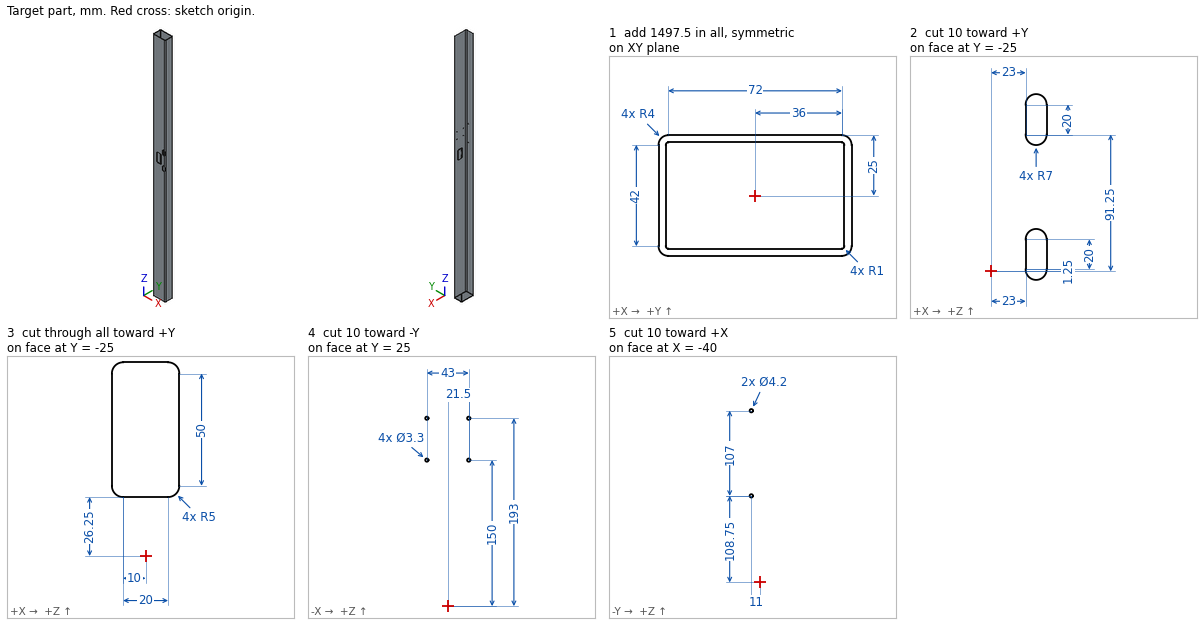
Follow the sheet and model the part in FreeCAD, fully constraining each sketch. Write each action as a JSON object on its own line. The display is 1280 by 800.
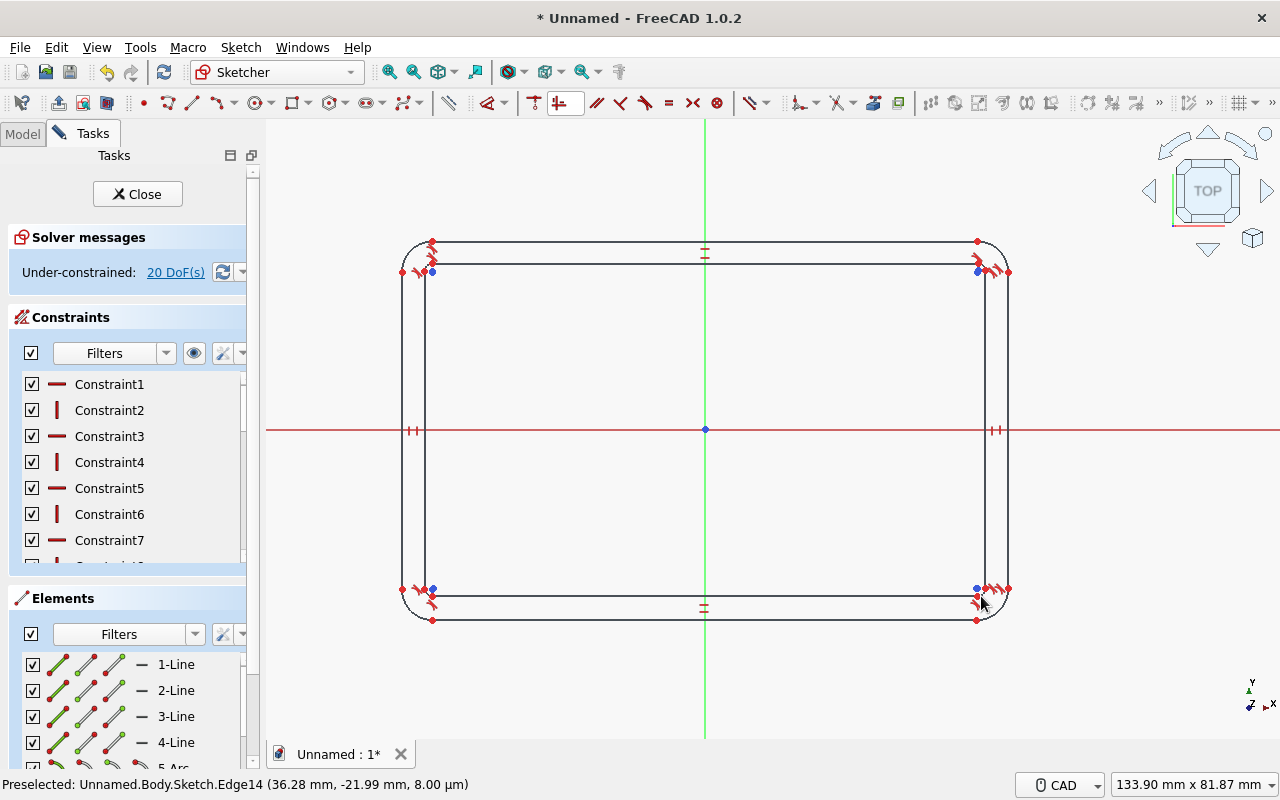
{"action": "left_click", "coordinate": [814, 596]}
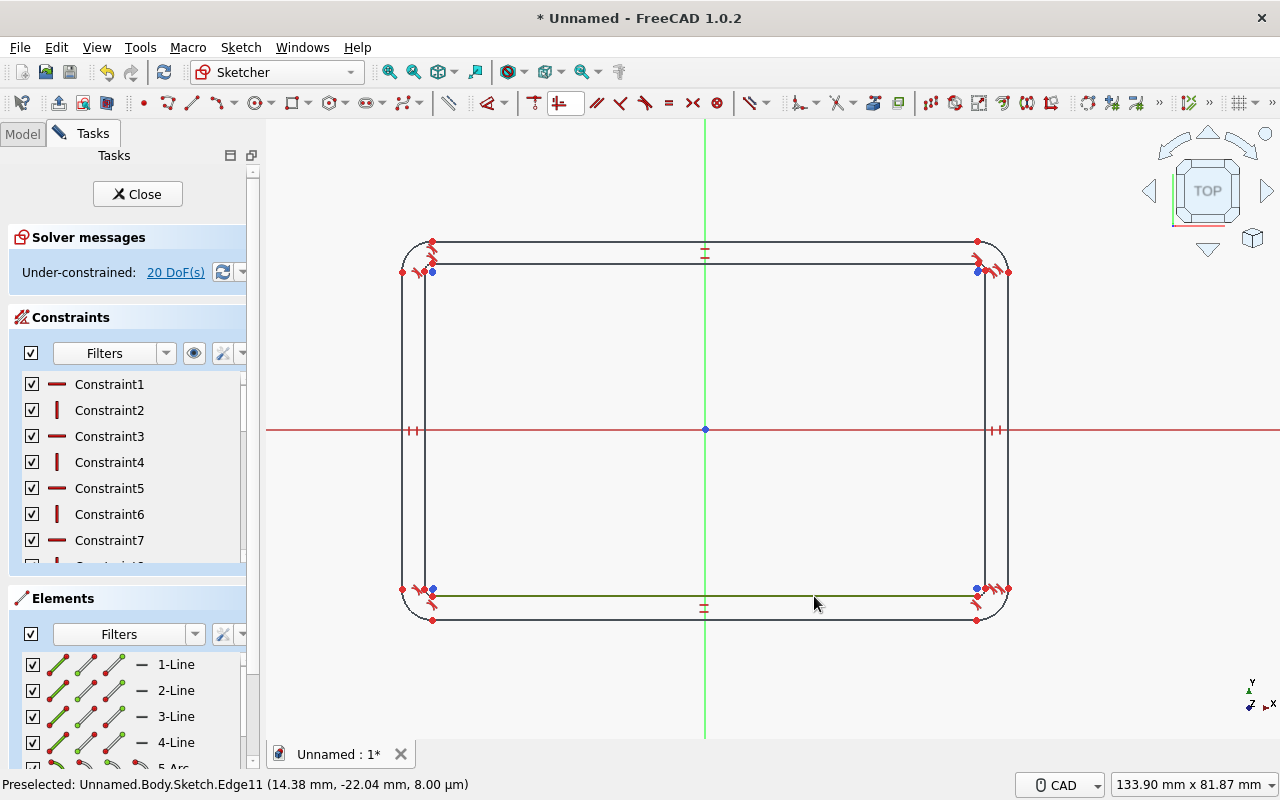
{"action": "scroll", "coordinate": [983, 594], "scroll_direction": "up", "scroll_amount": 5}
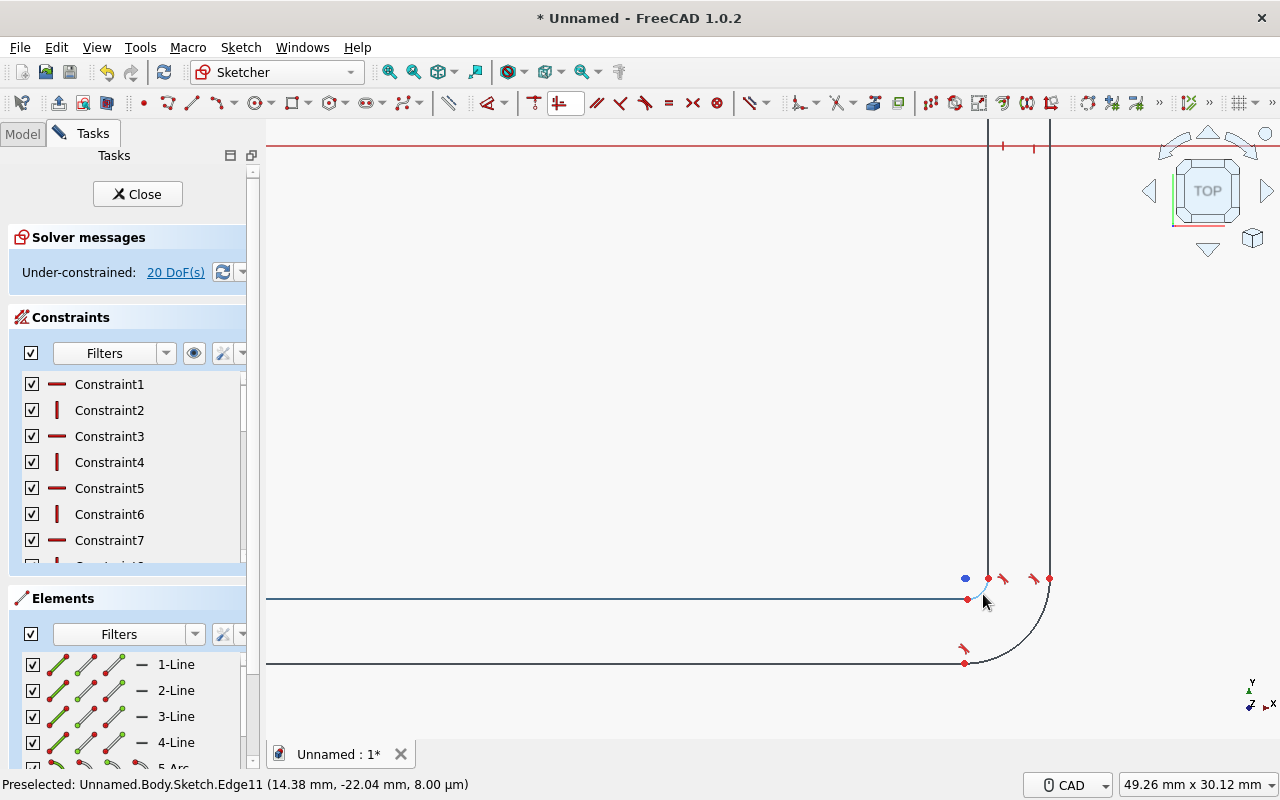
{"action": "left_click", "coordinate": [982, 593]}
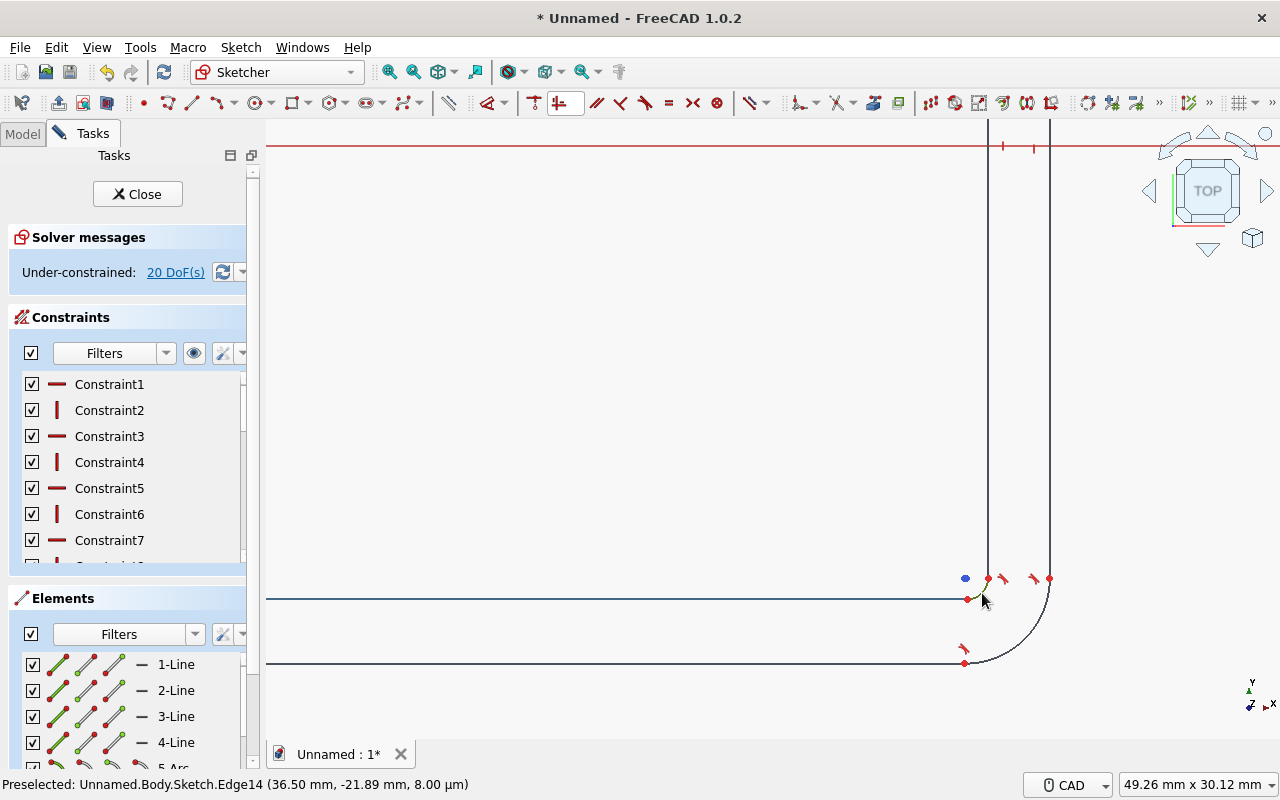
{"action": "key", "text": "t"}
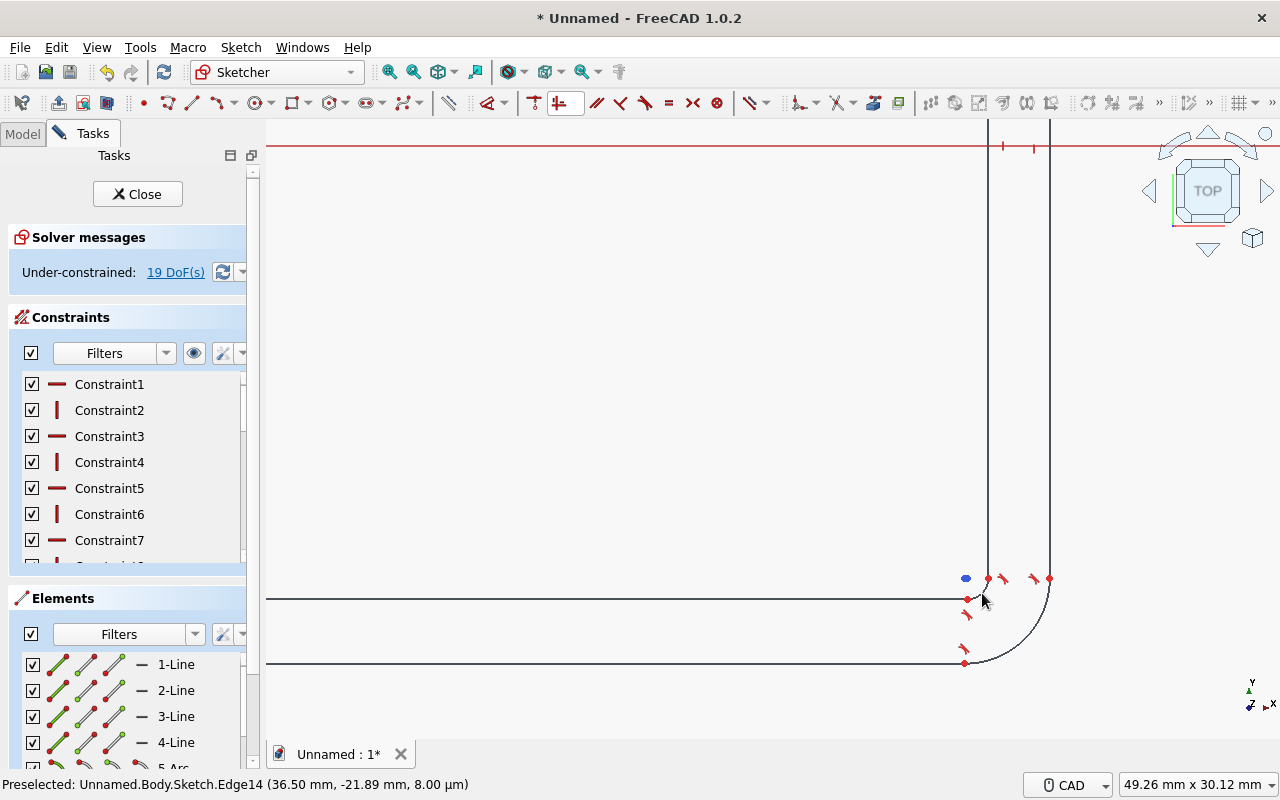
{"action": "left_click", "coordinate": [522, 599]}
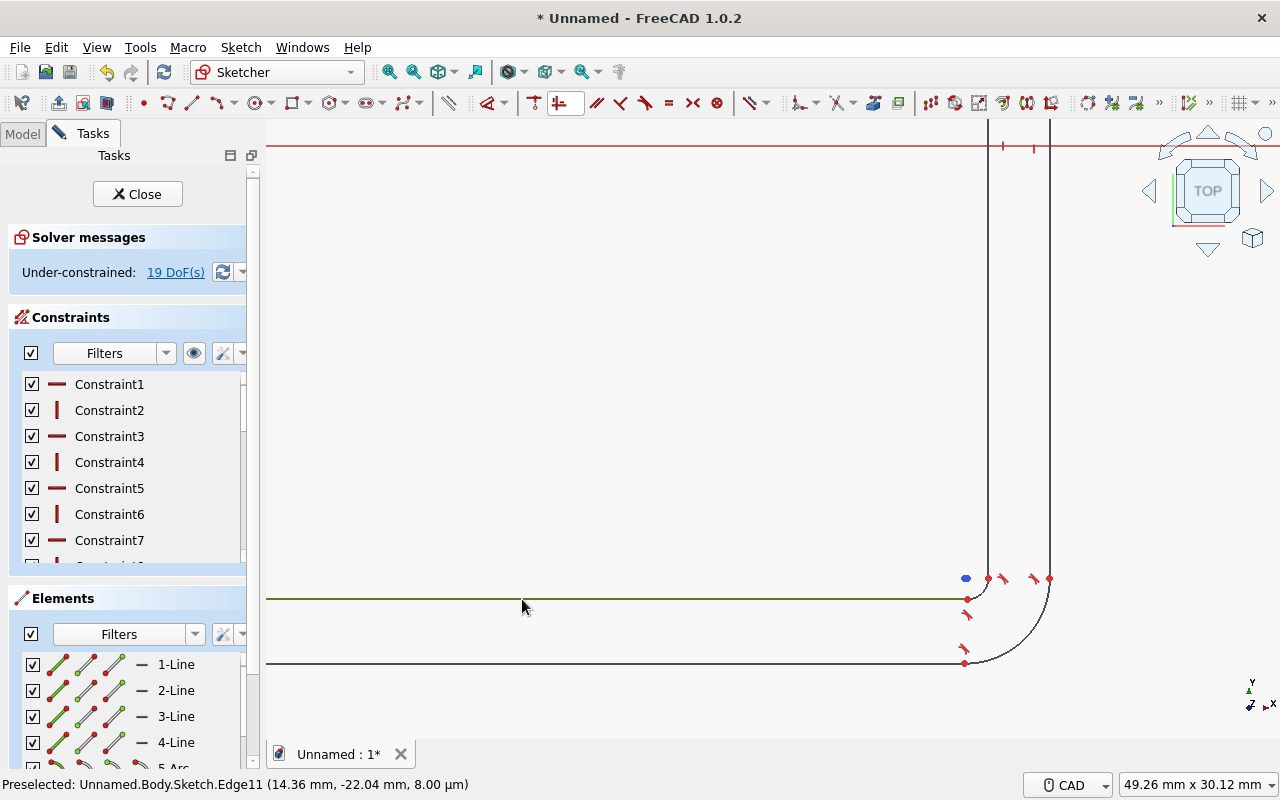
{"action": "scroll", "coordinate": [983, 594], "scroll_direction": "down", "scroll_amount": 5}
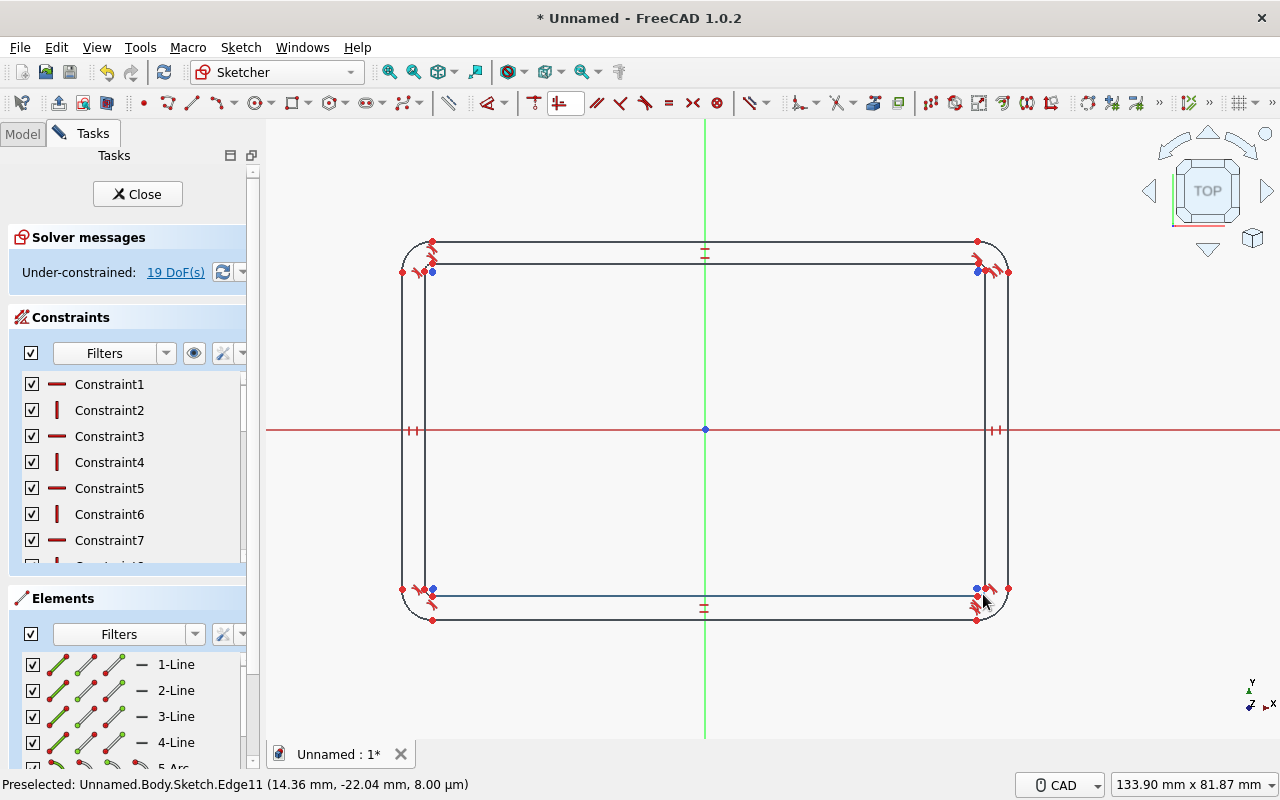
{"action": "scroll", "coordinate": [426, 592], "scroll_direction": "up", "scroll_amount": 8}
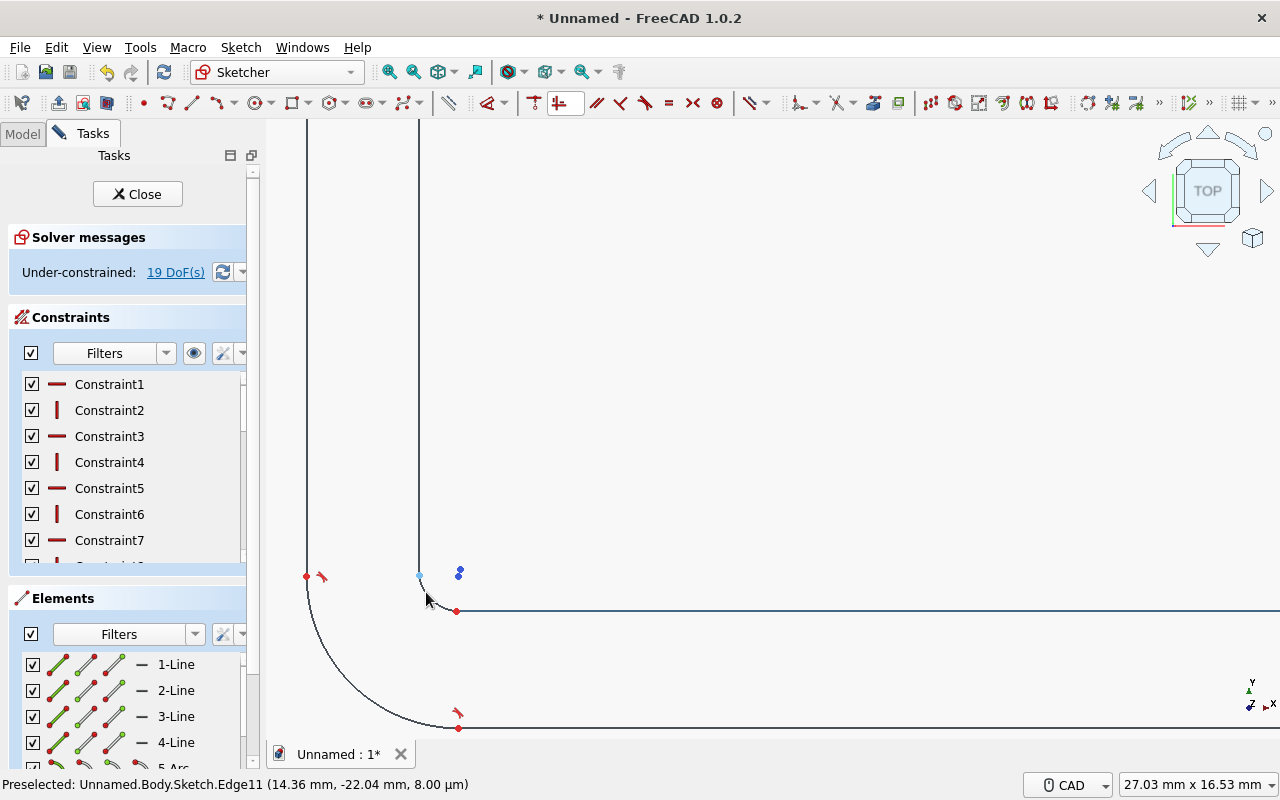
{"action": "left_click", "coordinate": [425, 591]}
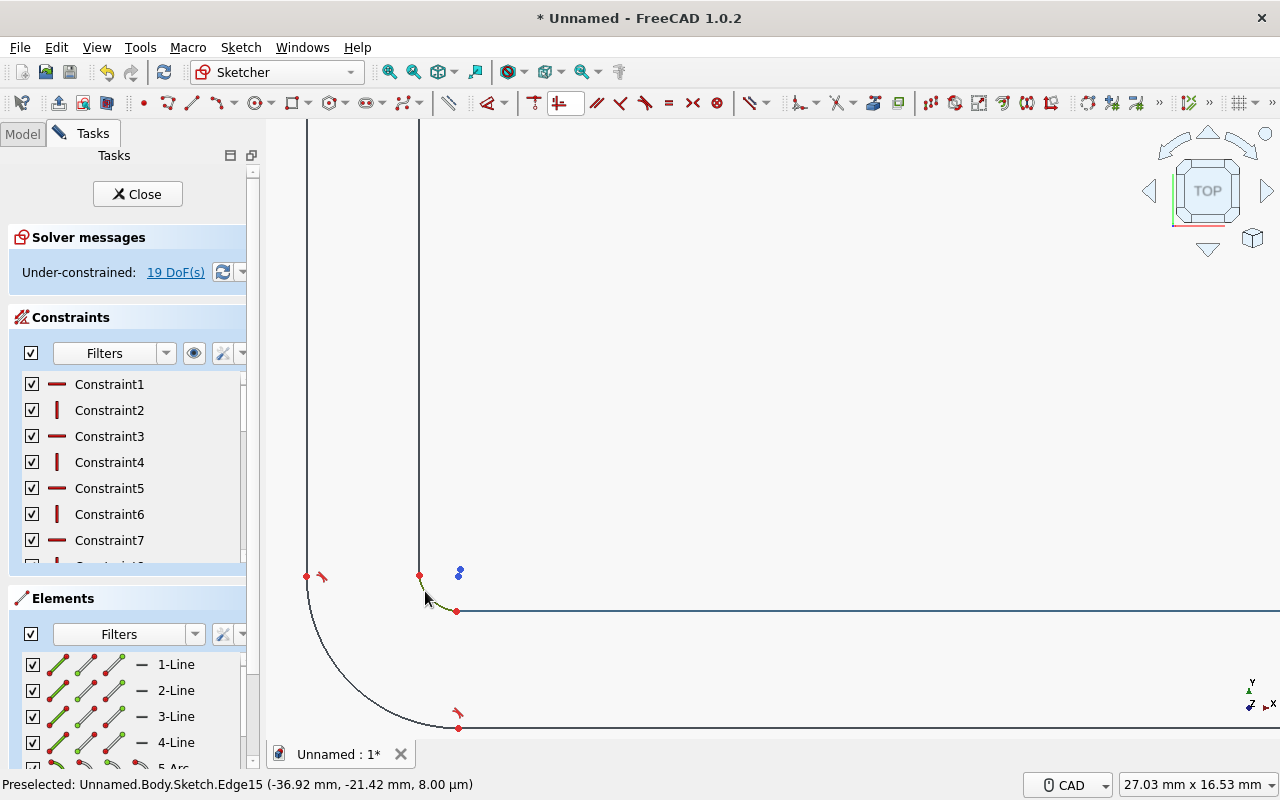
{"action": "left_click", "coordinate": [646, 104]}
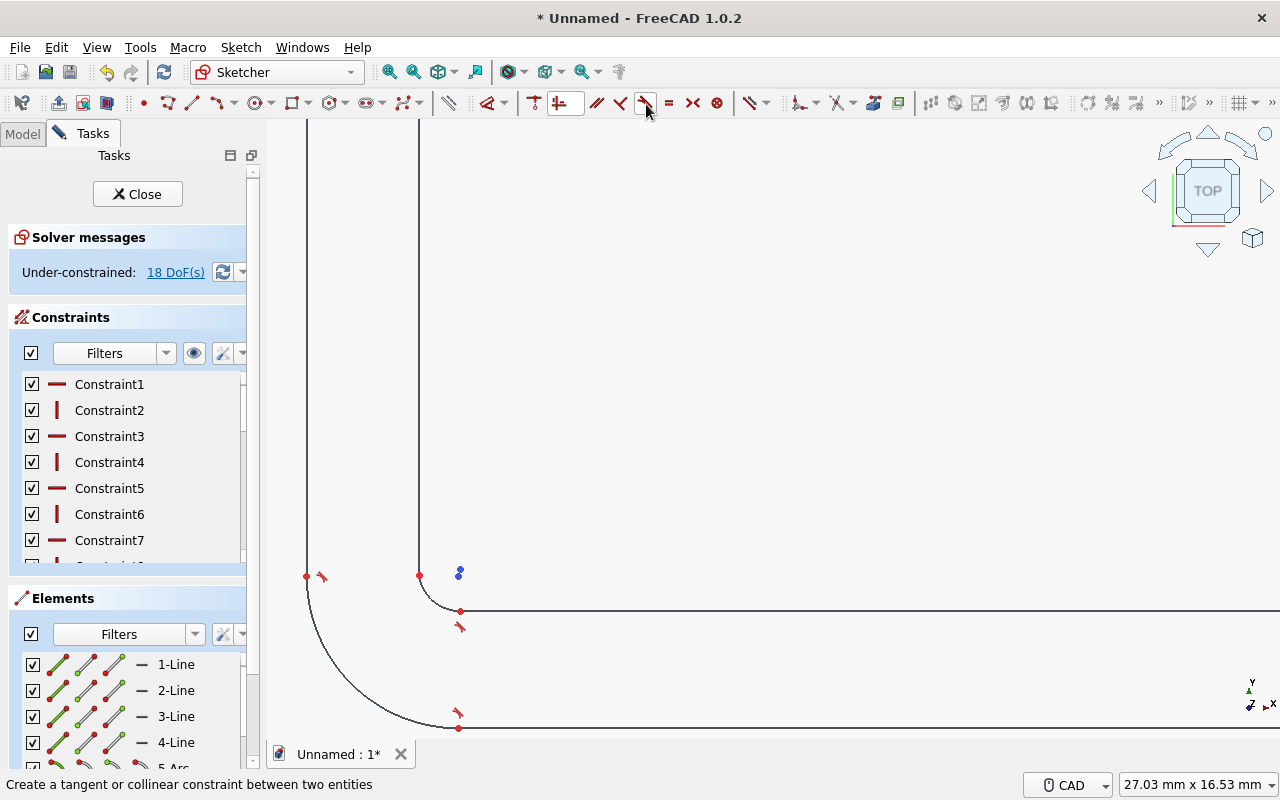
{"action": "scroll", "coordinate": [425, 592], "scroll_direction": "down", "scroll_amount": 8}